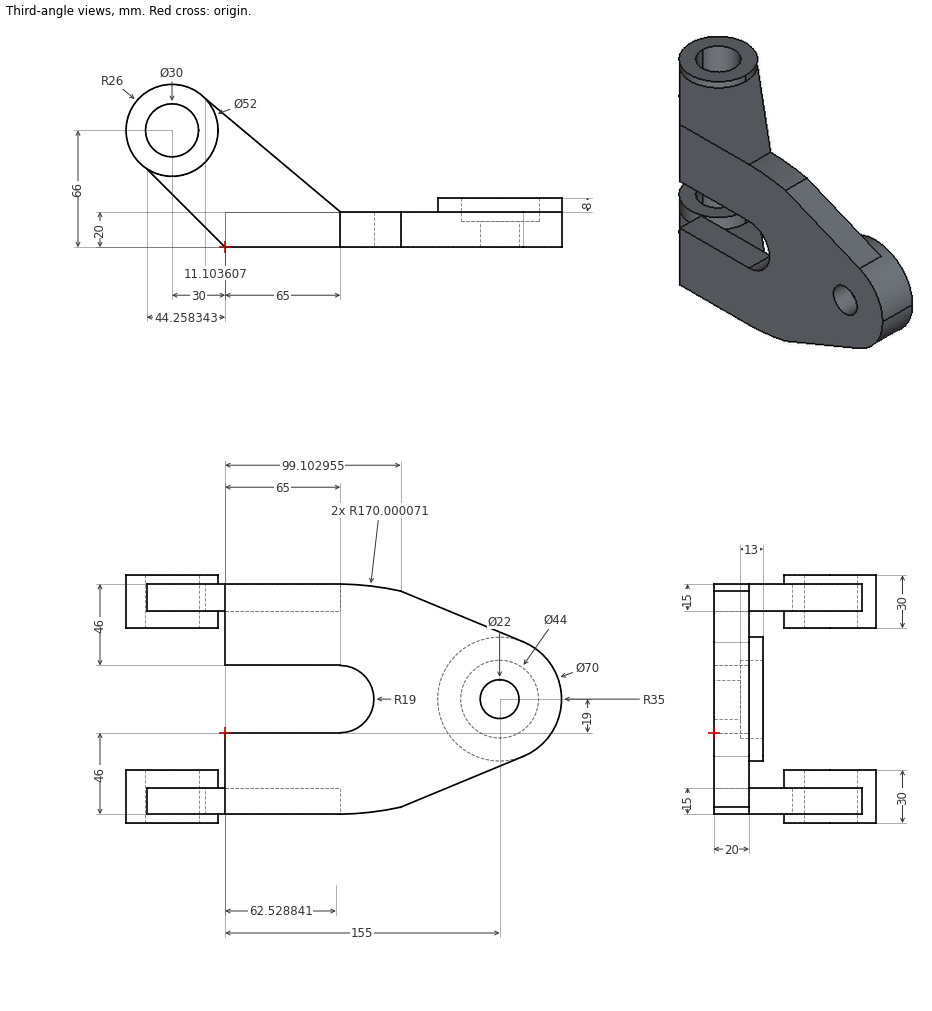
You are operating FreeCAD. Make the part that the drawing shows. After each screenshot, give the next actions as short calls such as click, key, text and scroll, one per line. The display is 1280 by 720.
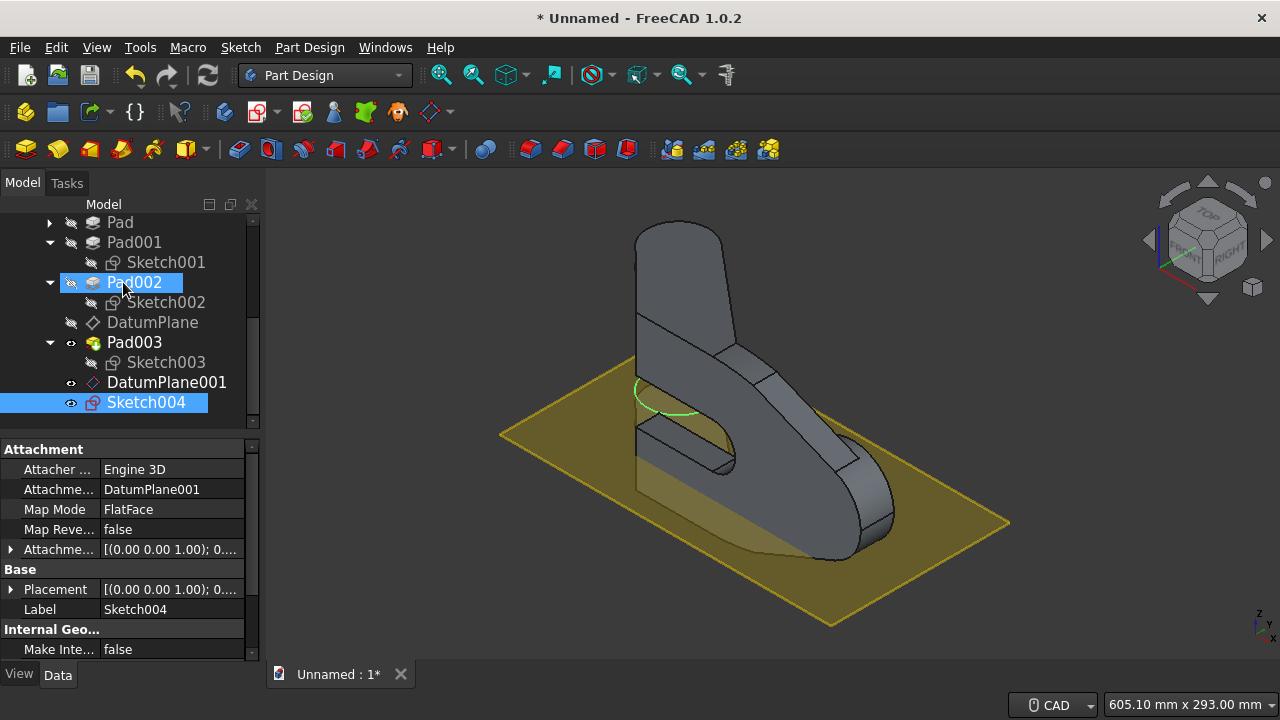
click(26, 150)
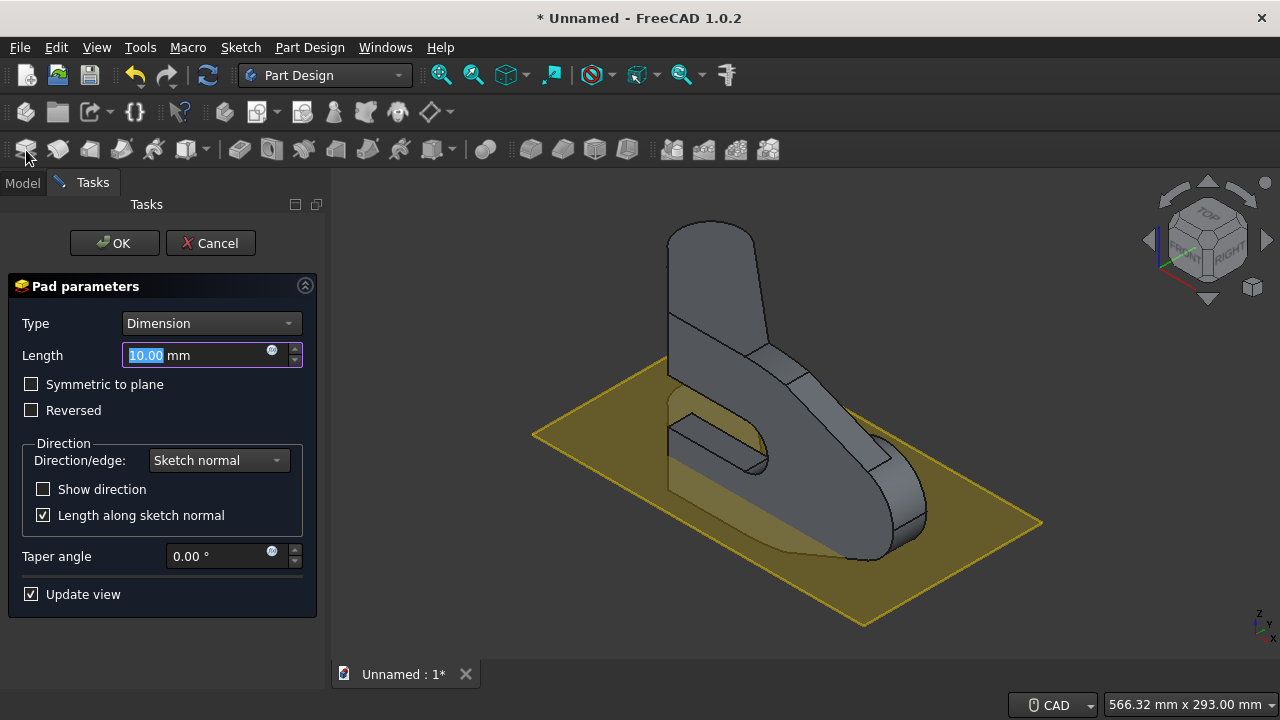
text(30)
key(Tab)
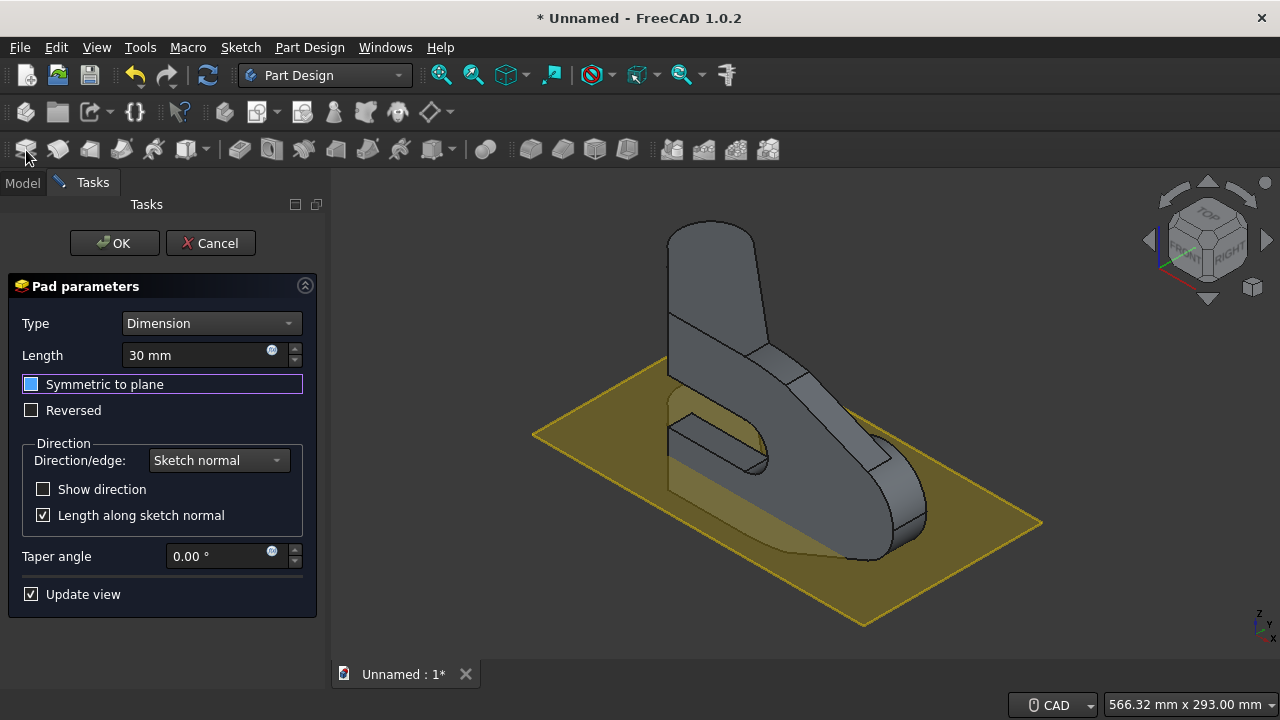
click(30, 410)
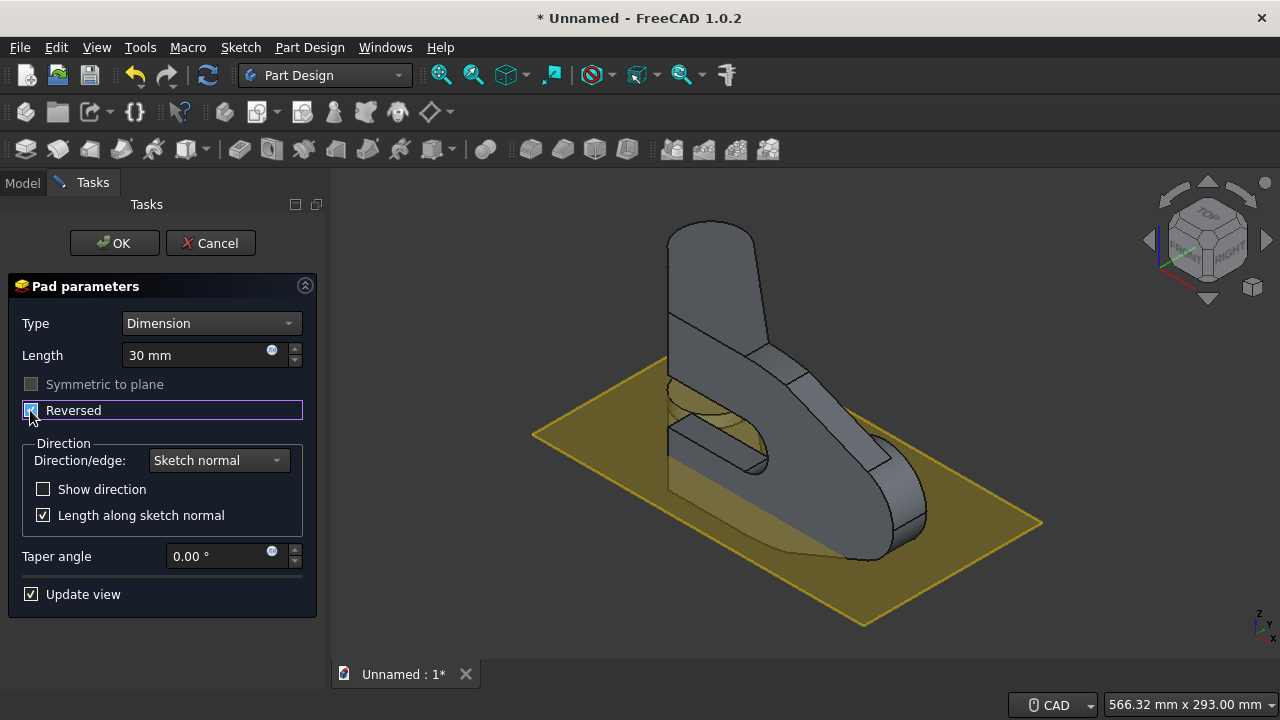
click(115, 243)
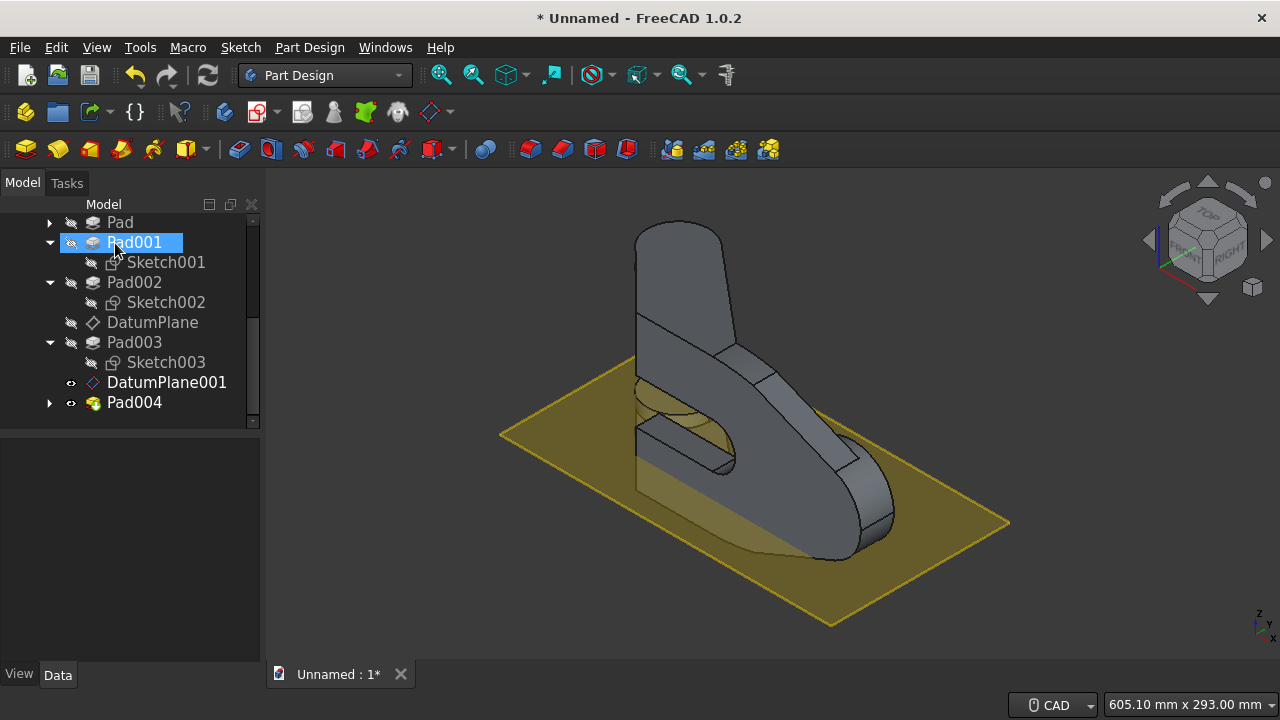
click(116, 383)
key(space)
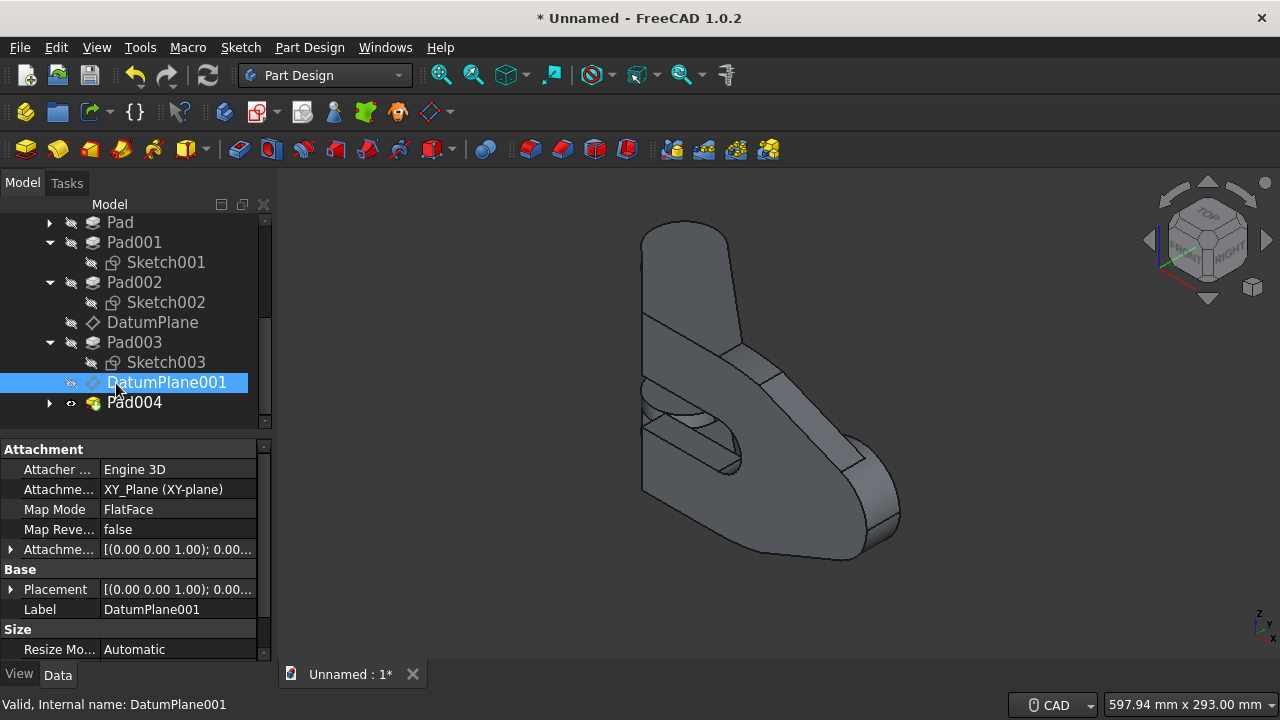
scroll(140, 318, down, 3)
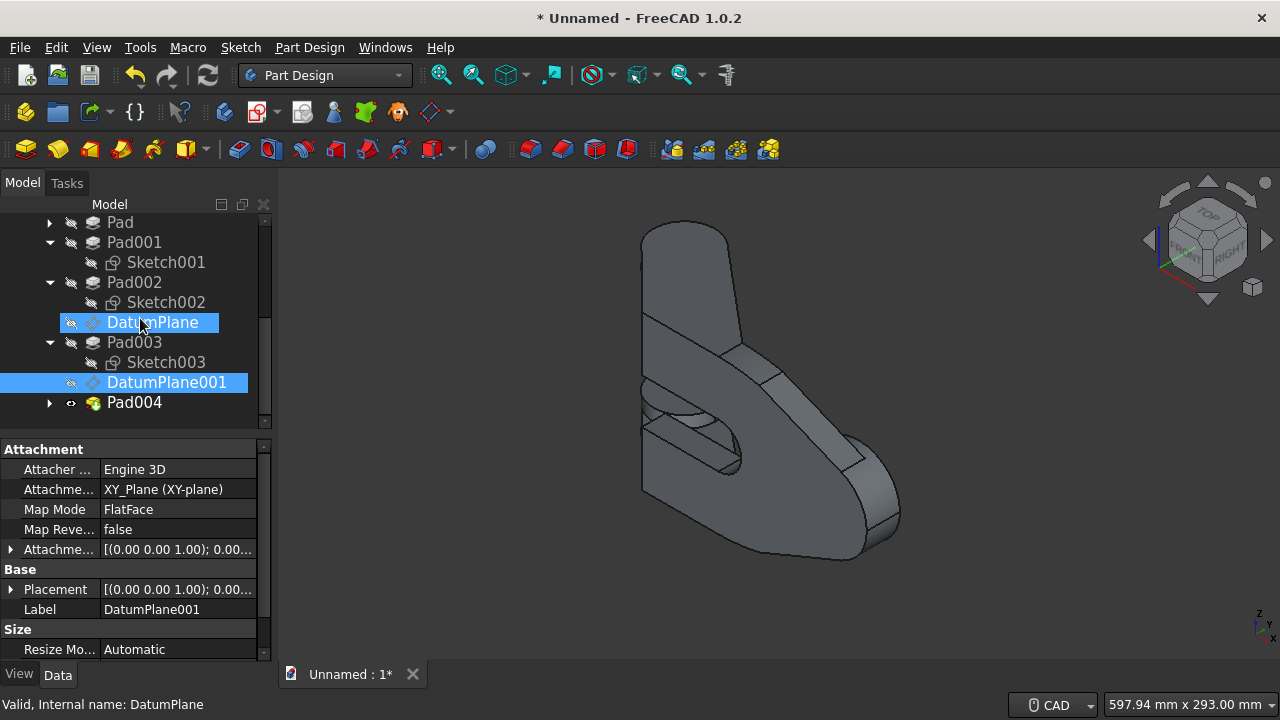
scroll(140, 318, up, 15)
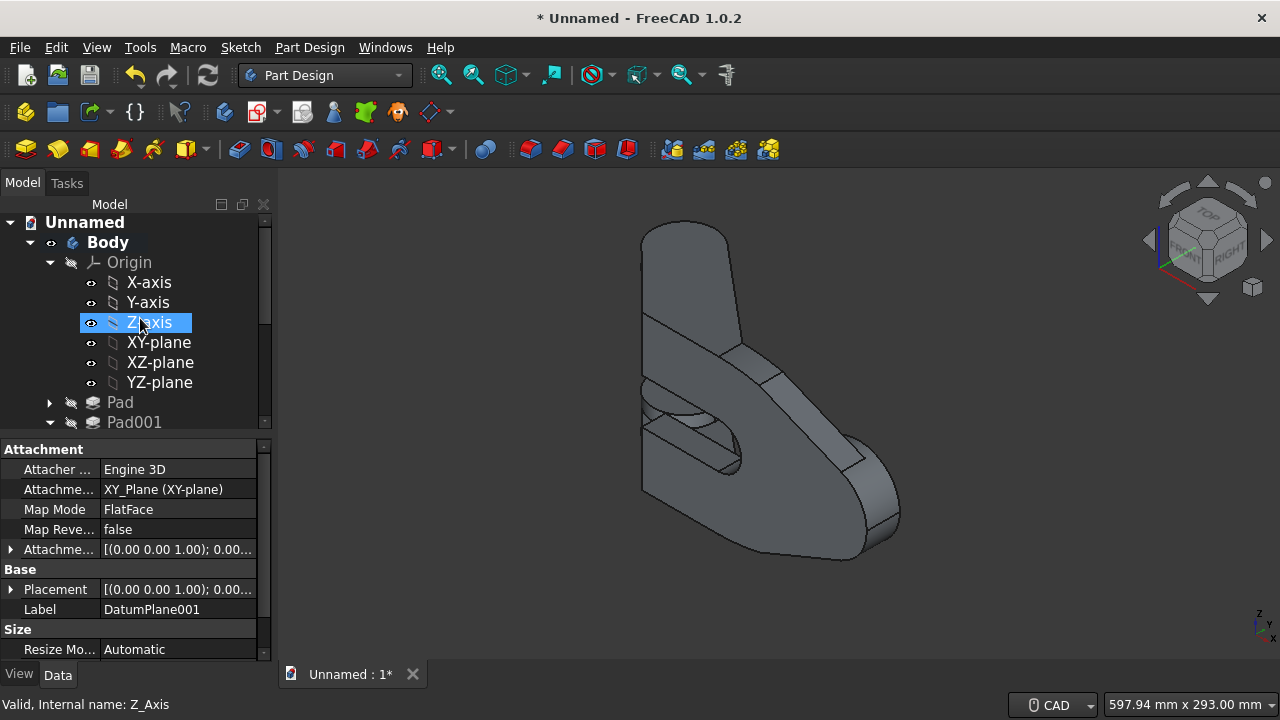
click(136, 343)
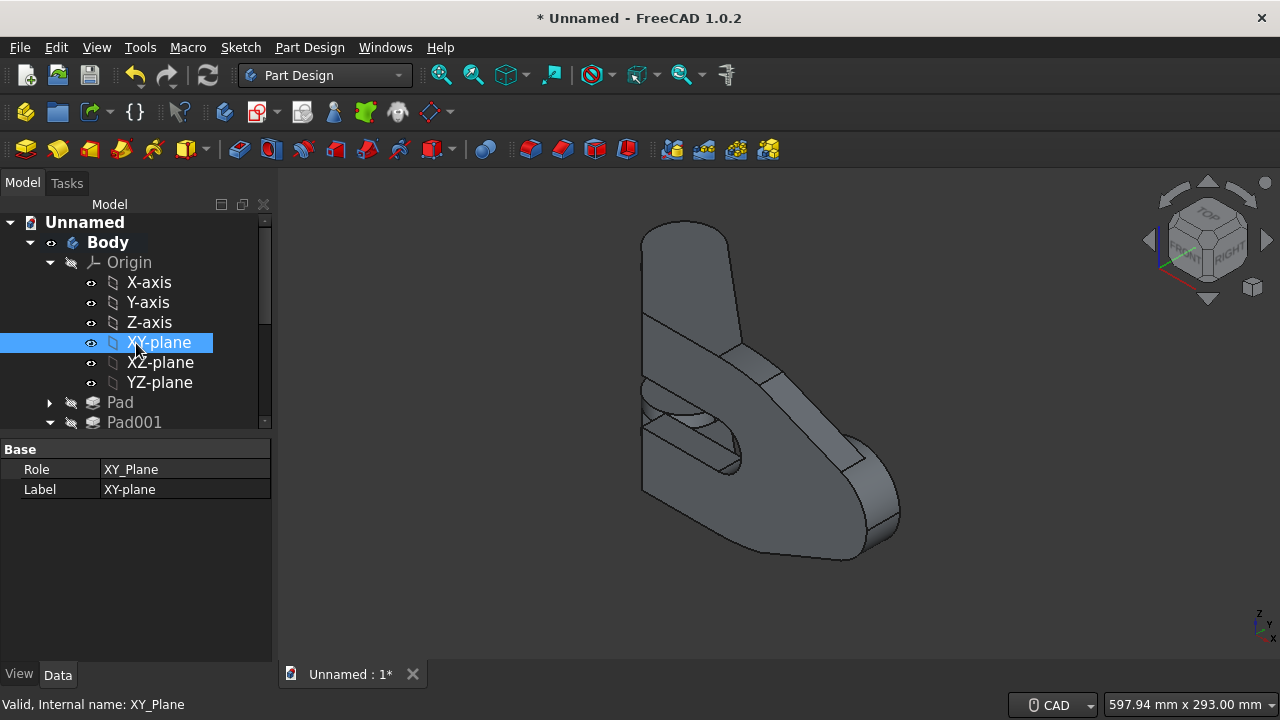
click(430, 112)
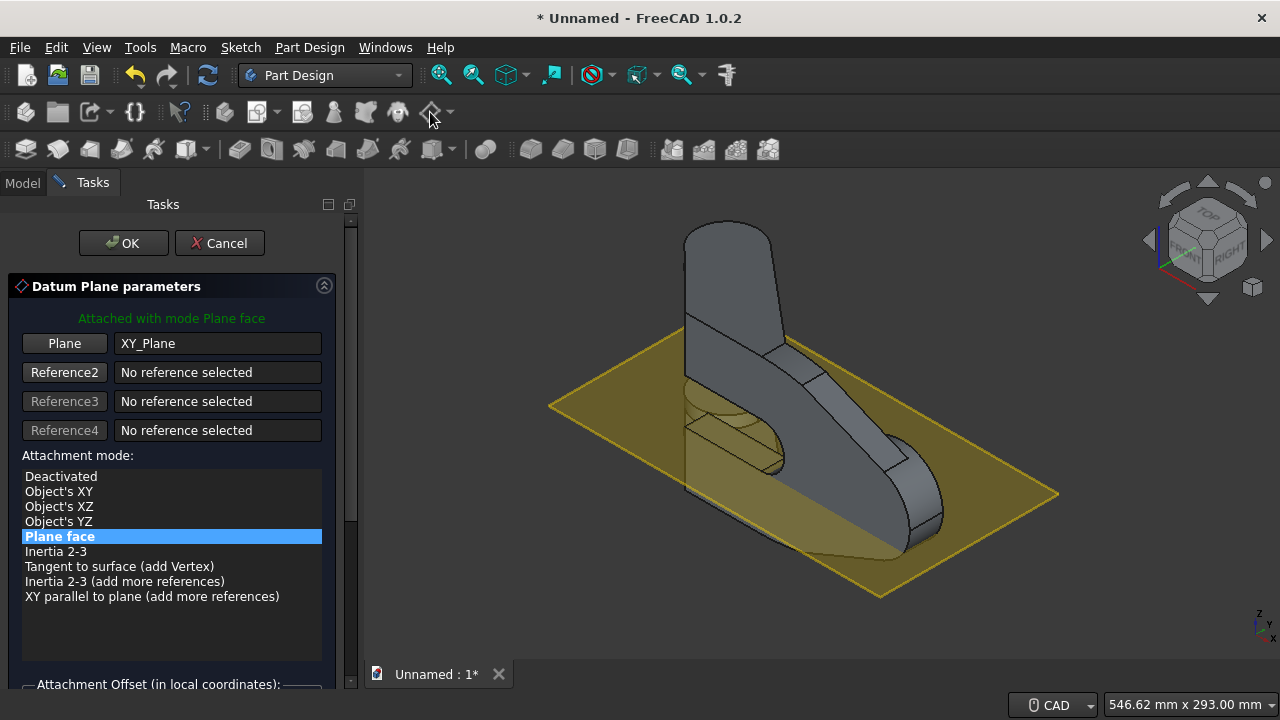
scroll(351, 451, down, 3)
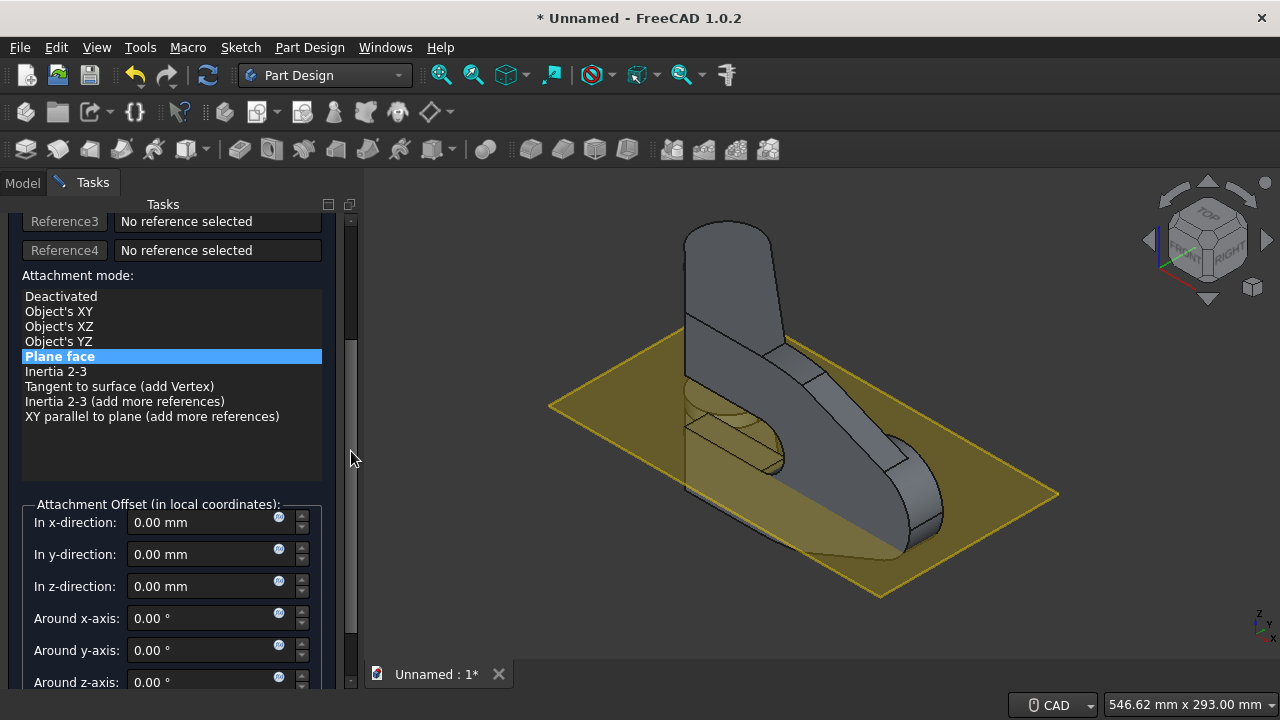
triple_click(210, 586)